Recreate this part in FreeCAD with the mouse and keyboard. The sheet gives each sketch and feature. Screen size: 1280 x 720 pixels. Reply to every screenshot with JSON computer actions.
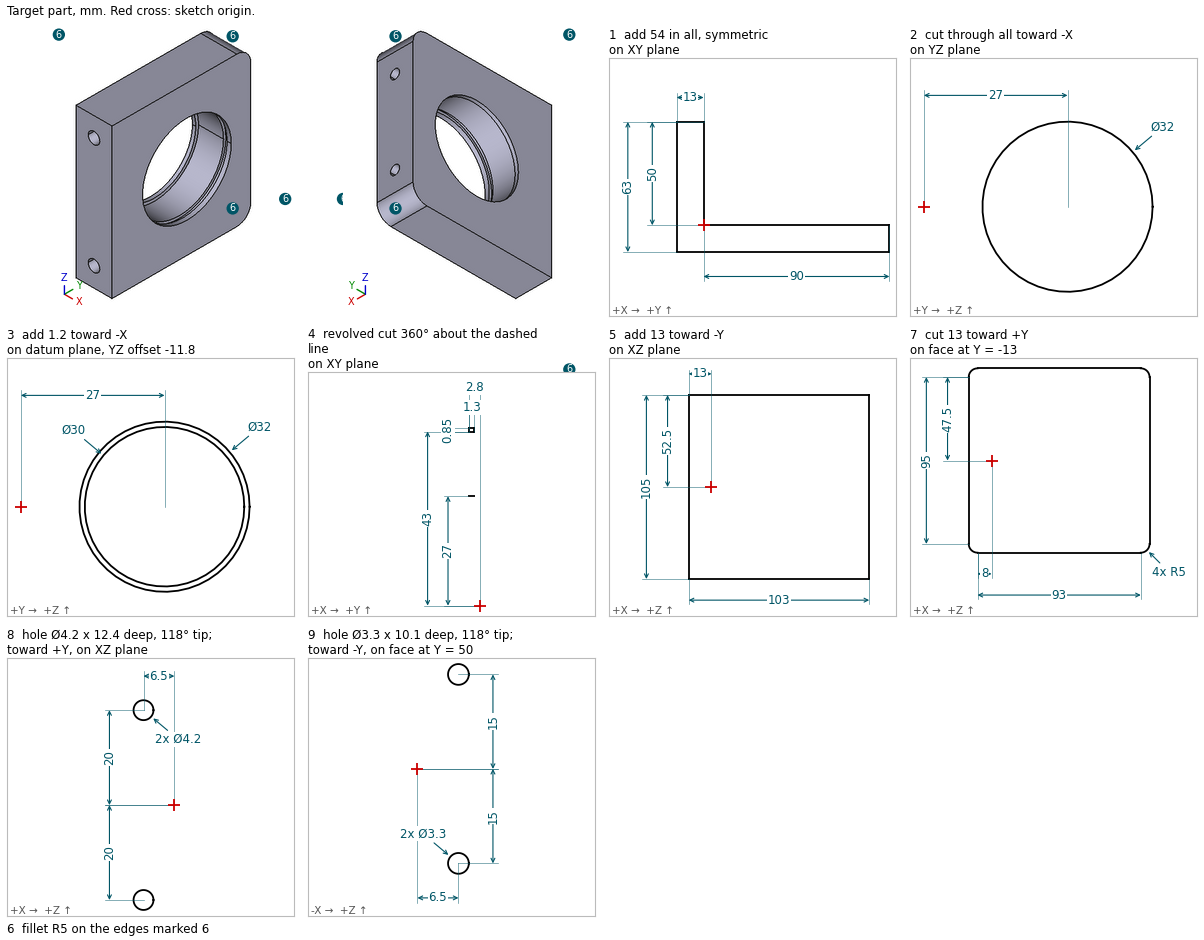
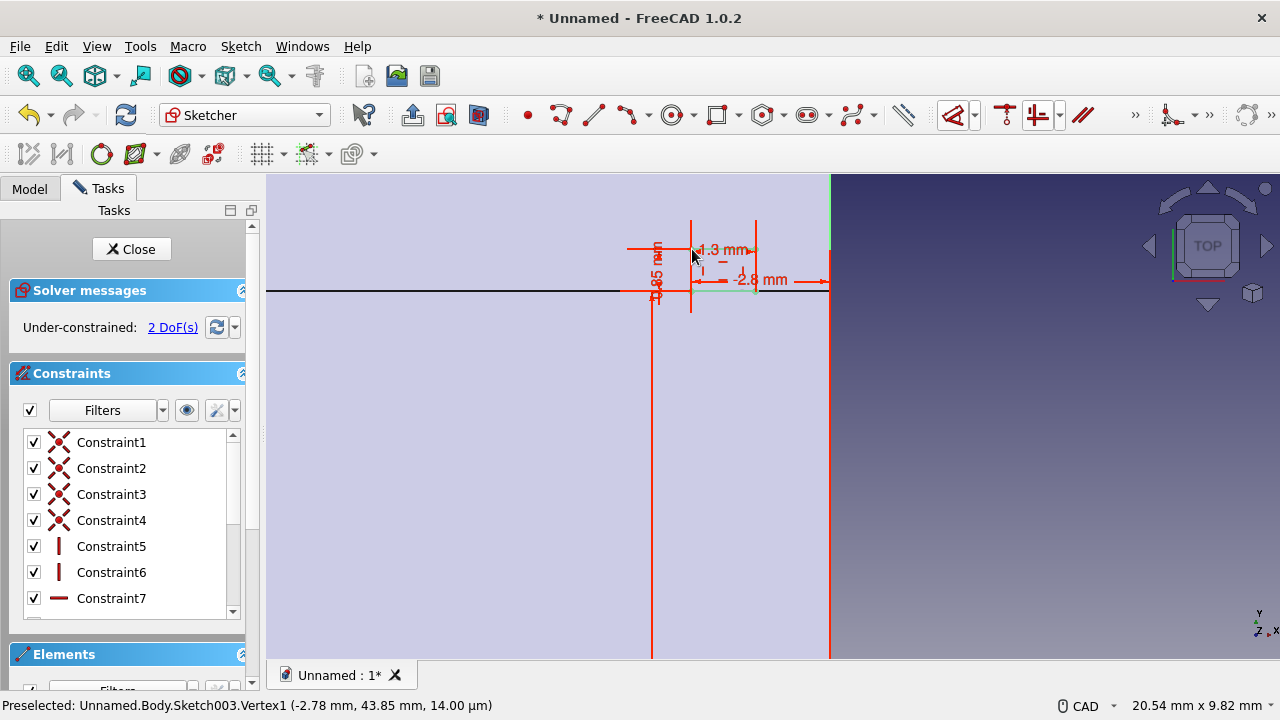
{"action": "left_click", "coordinate": [132, 249]}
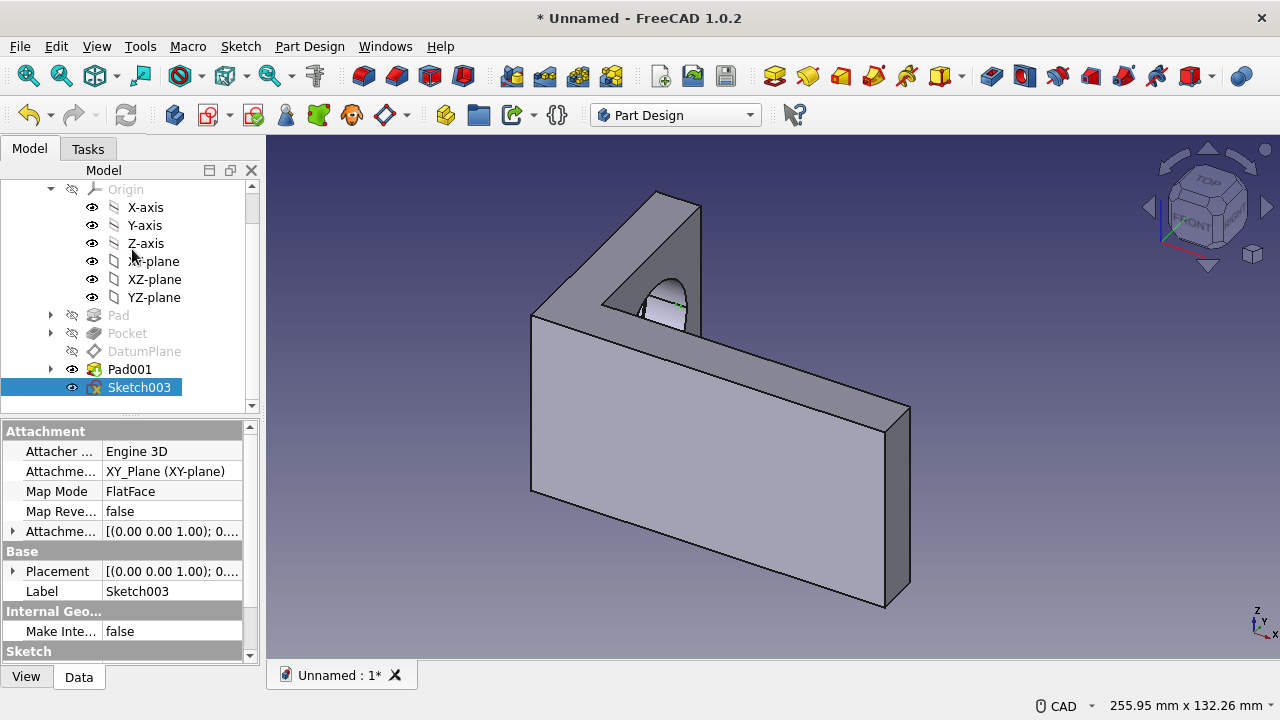
{"action": "left_click", "coordinate": [1058, 76]}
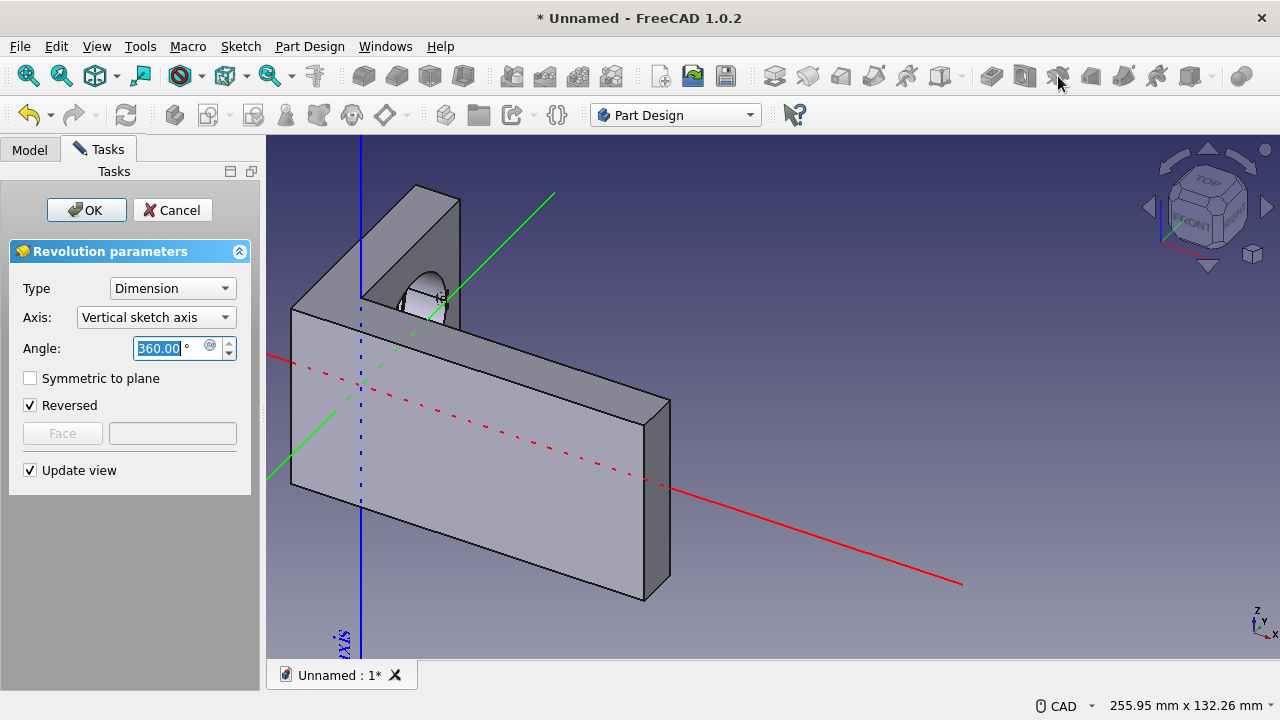
{"action": "left_click", "coordinate": [157, 318]}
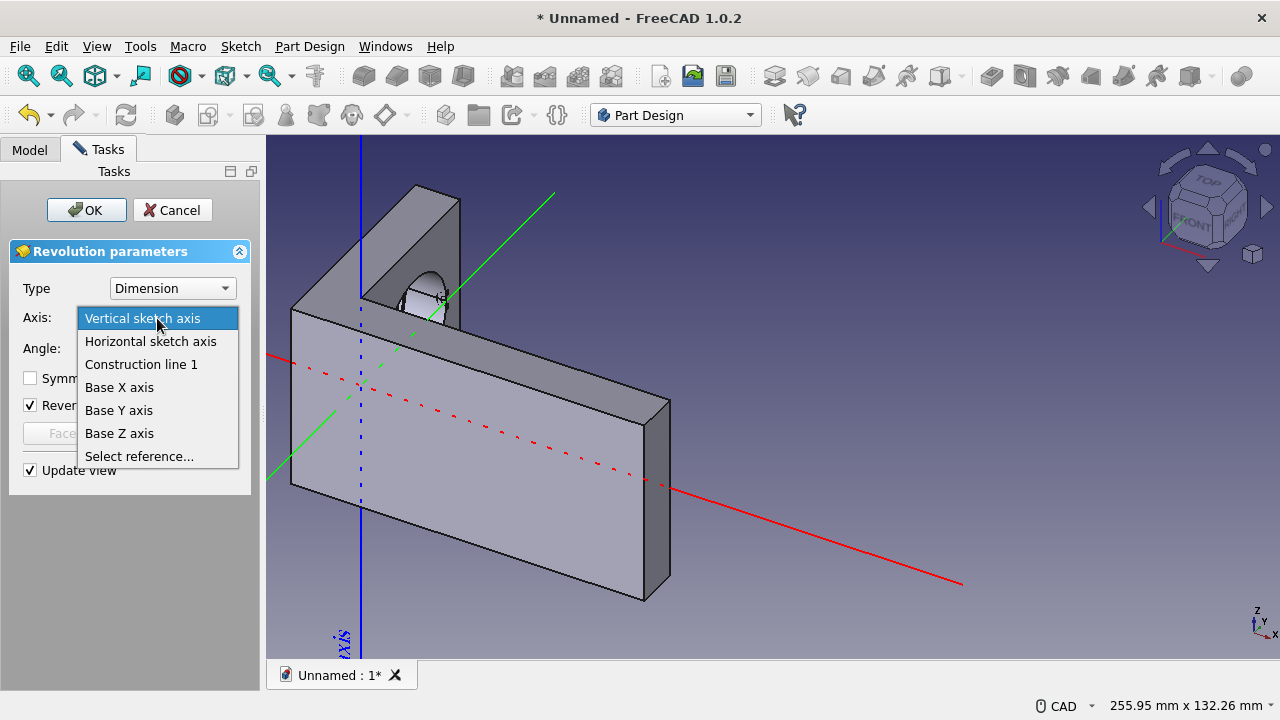
{"action": "left_click", "coordinate": [156, 364]}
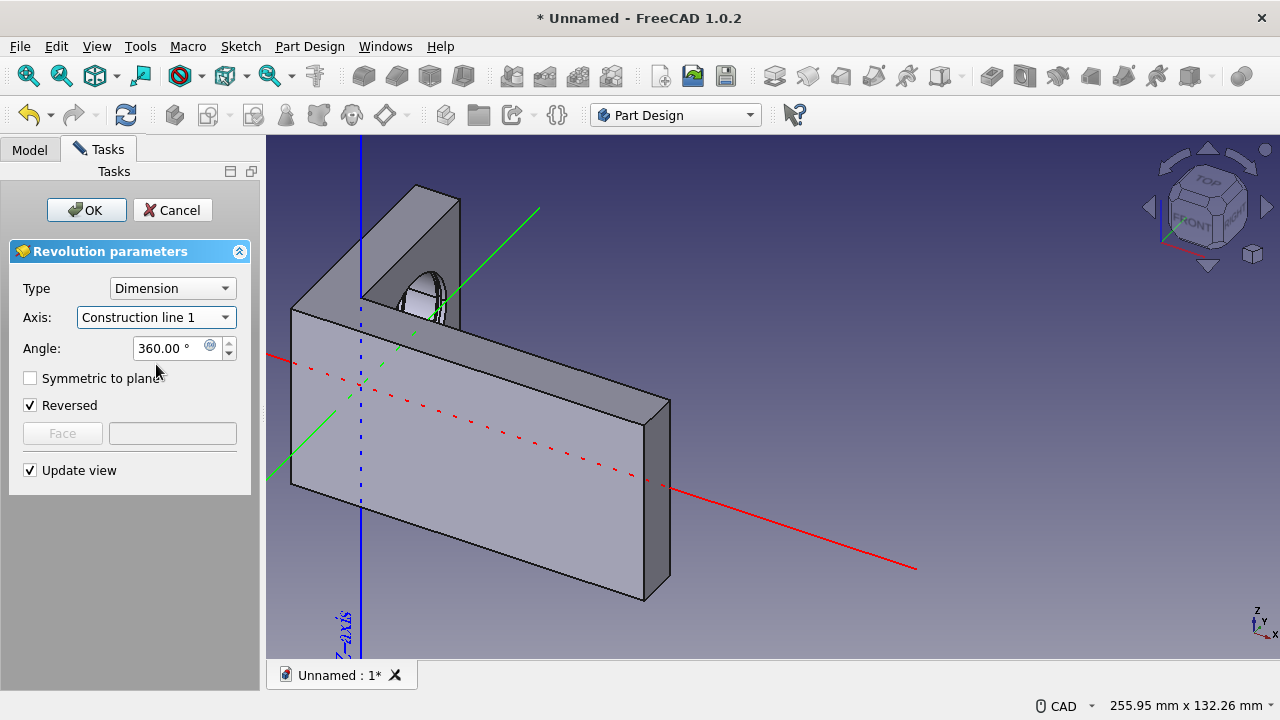
{"action": "left_click", "coordinate": [87, 210]}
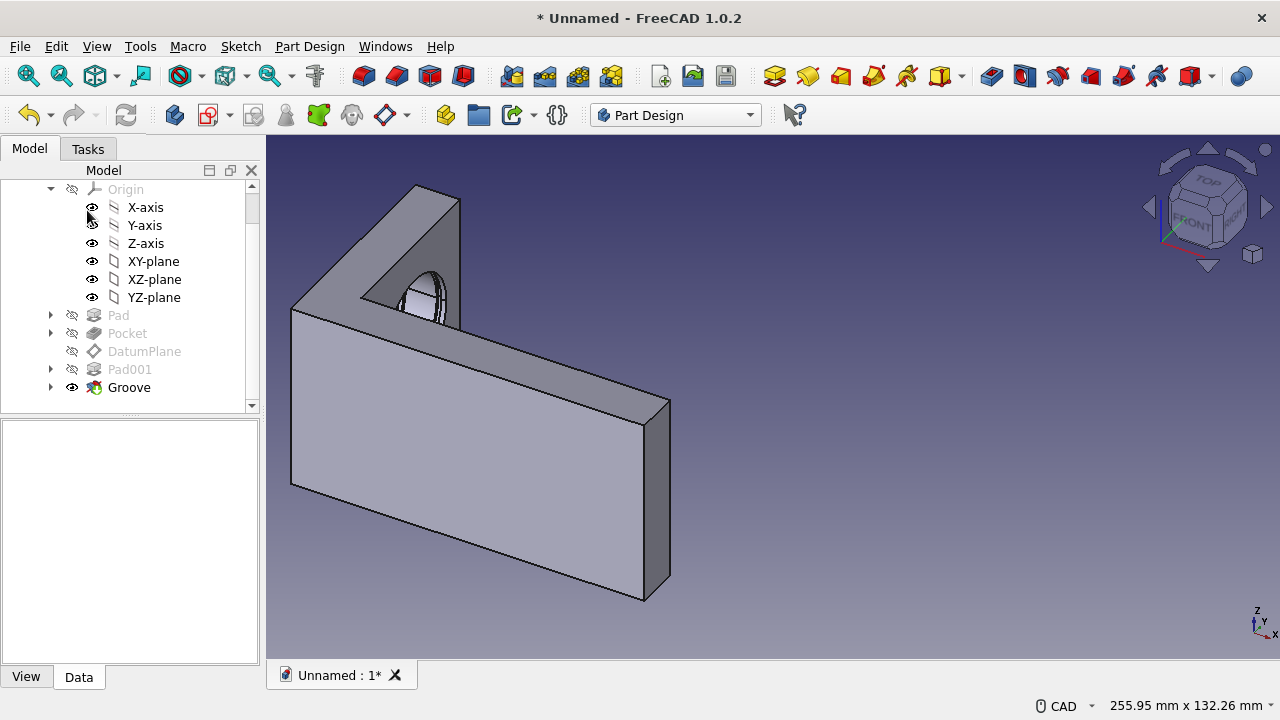
{"action": "left_click", "coordinate": [208, 116]}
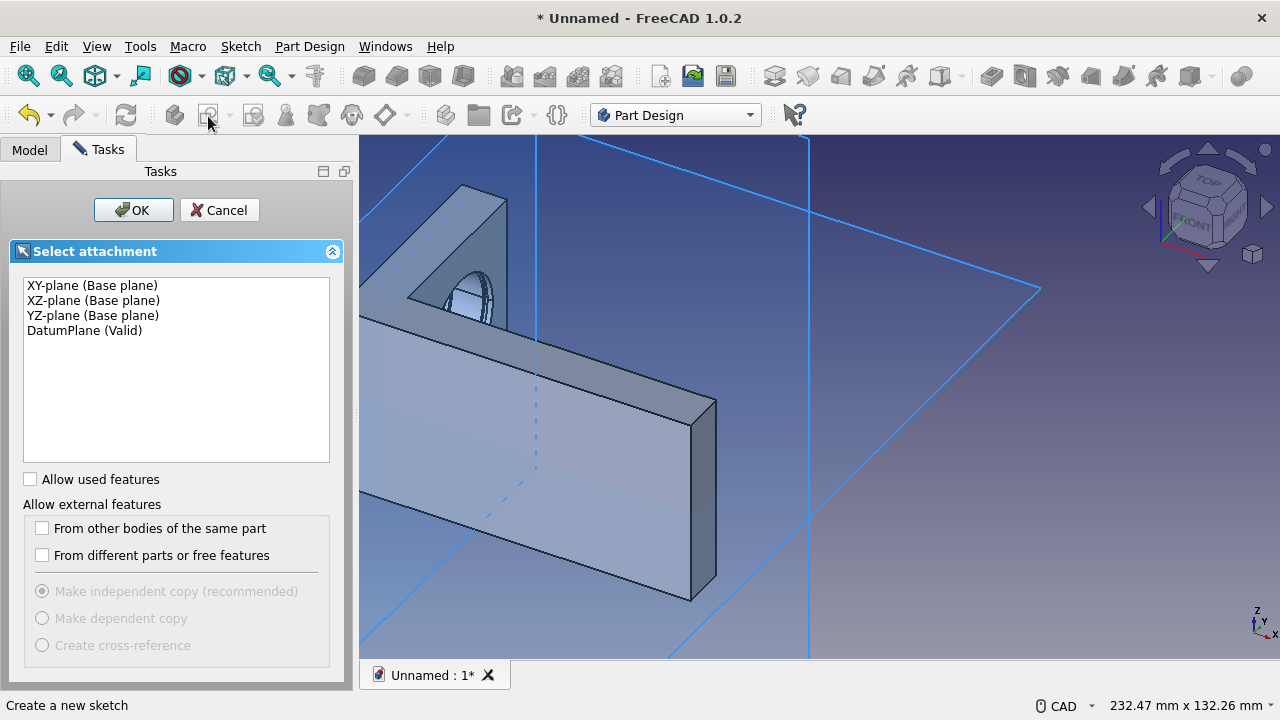
{"action": "left_click", "coordinate": [84, 300]}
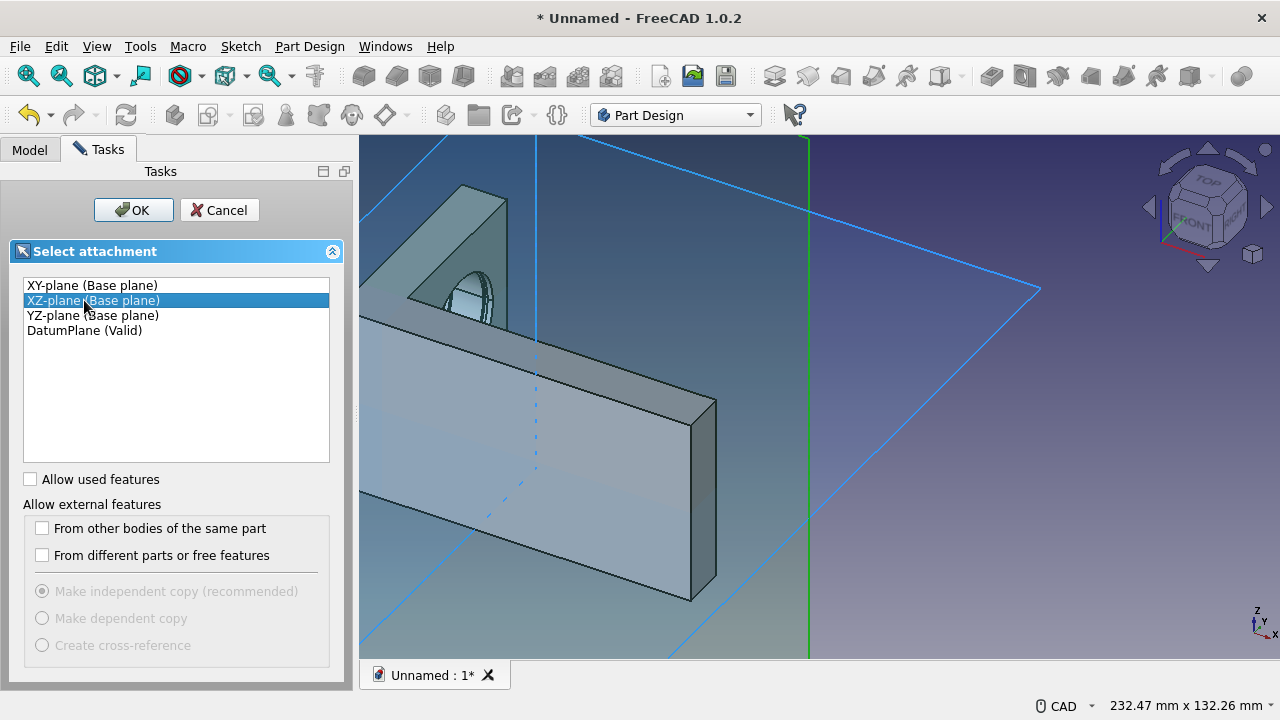
{"action": "left_click", "coordinate": [134, 210]}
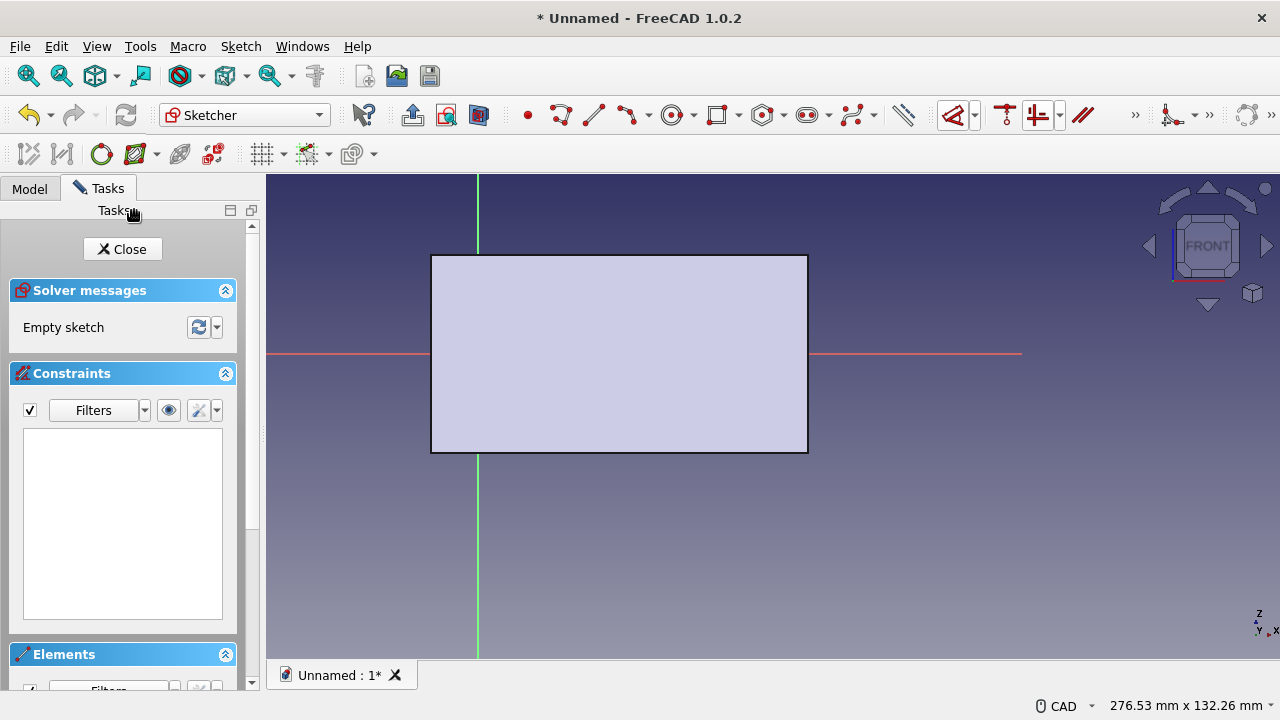
{"action": "left_click", "coordinate": [479, 116]}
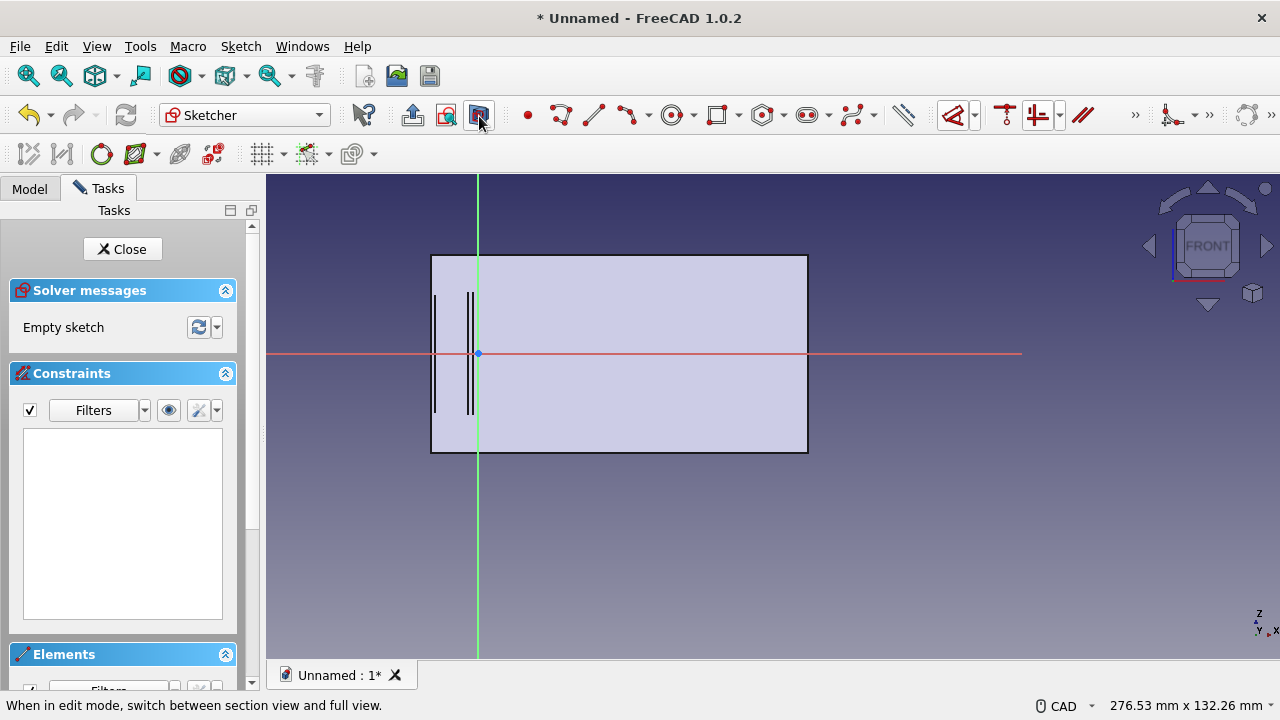
{"action": "scroll", "coordinate": [1088, 631], "scroll_direction": "down", "scroll_amount": 1}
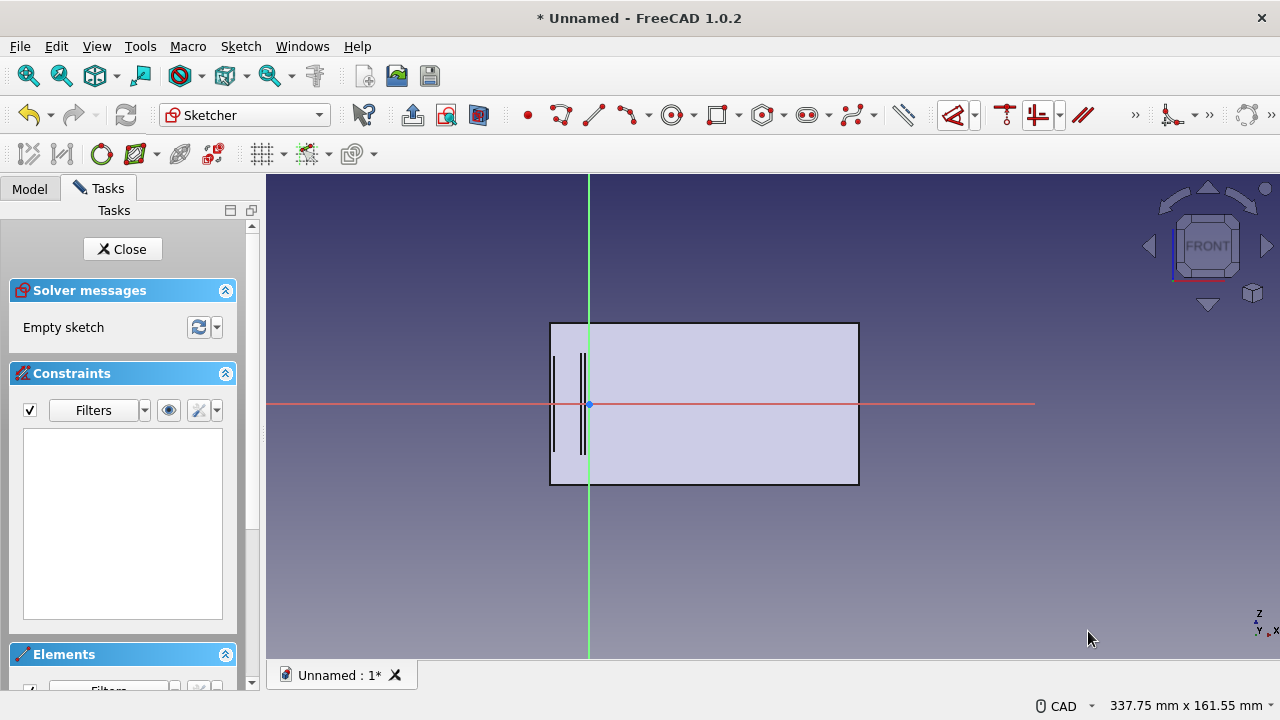
{"action": "left_click", "coordinate": [716, 116]}